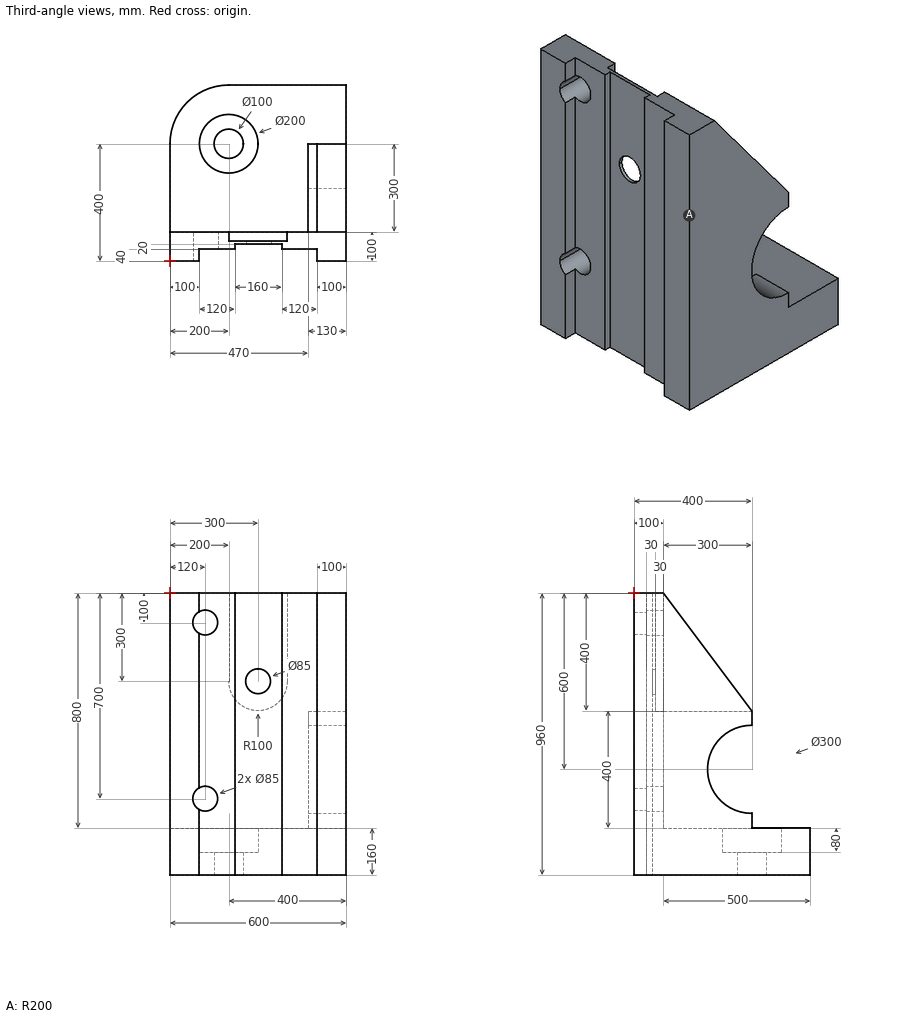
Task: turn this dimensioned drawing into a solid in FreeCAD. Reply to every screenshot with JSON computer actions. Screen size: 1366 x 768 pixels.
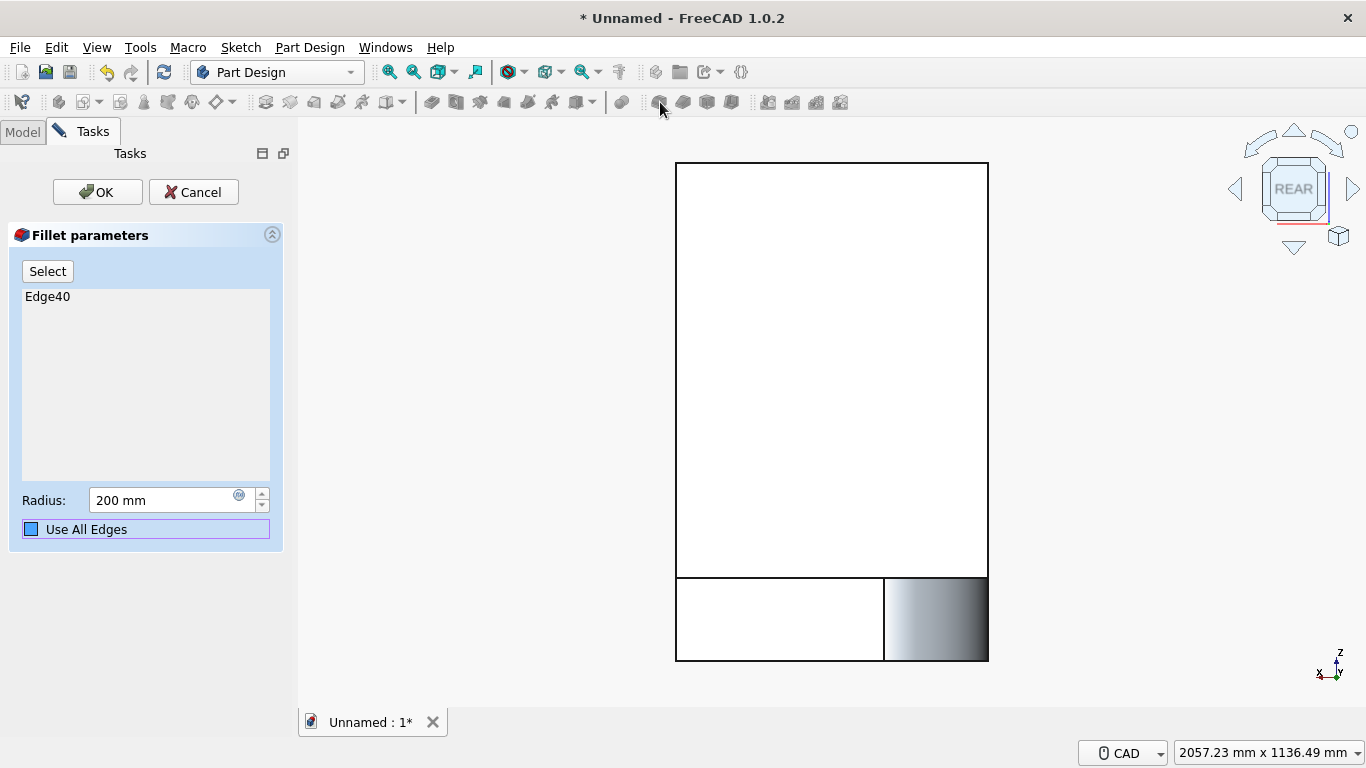
{"action": "left_click", "coordinate": [98, 192]}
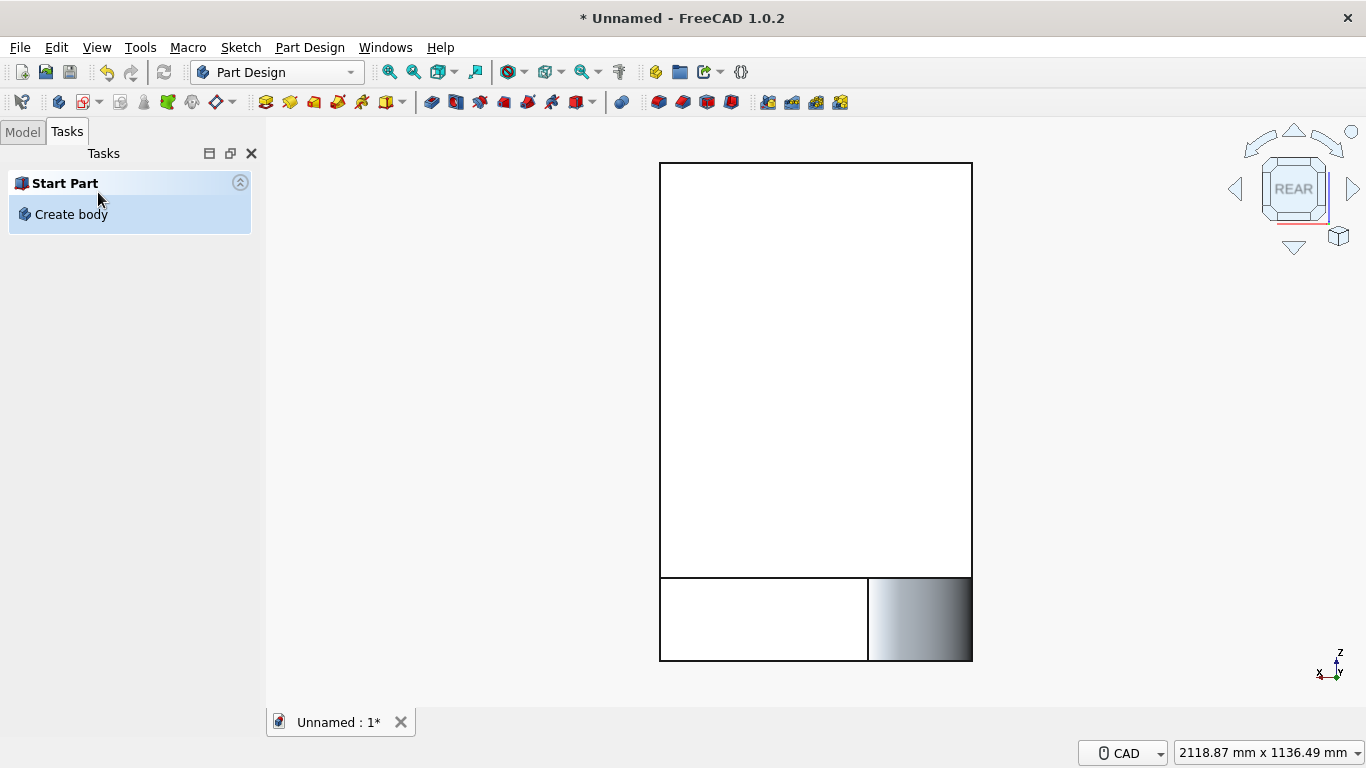
{"action": "key", "text": "0"}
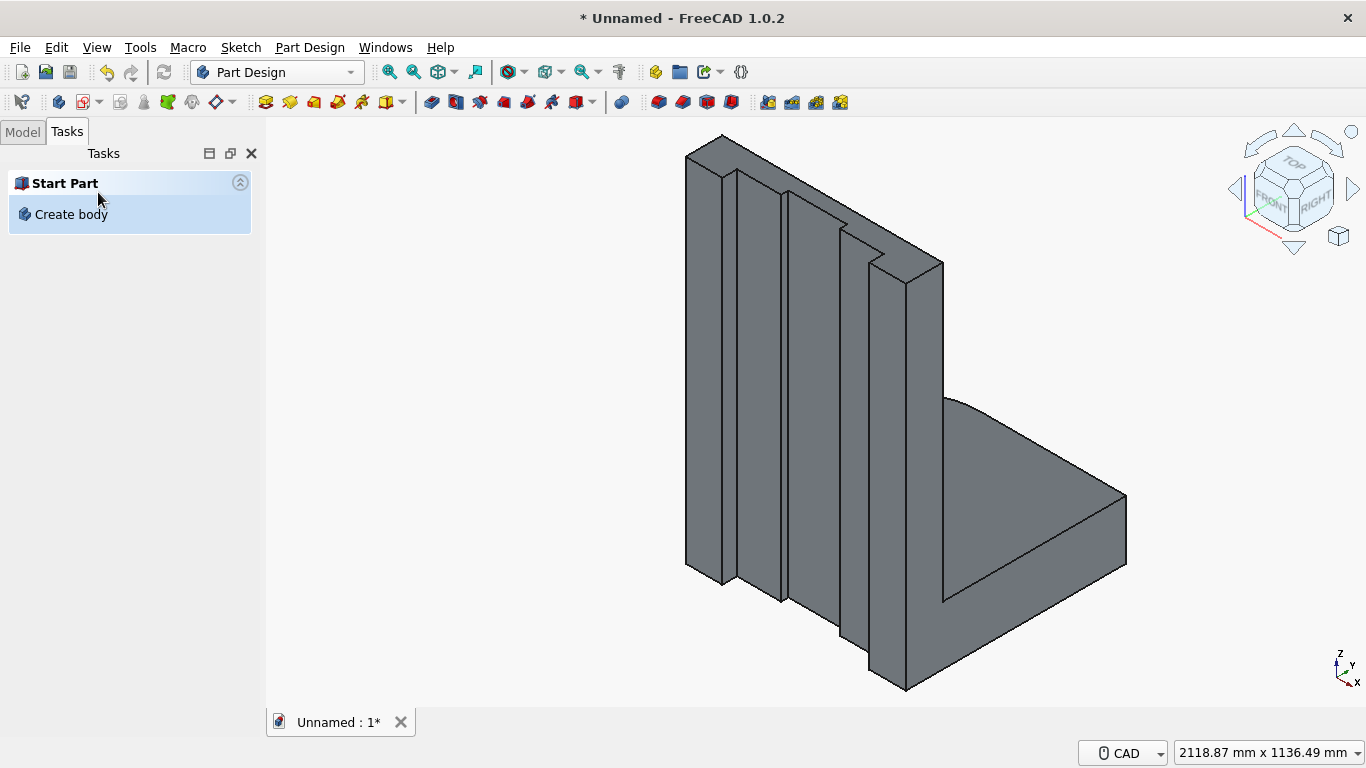
{"action": "left_click", "coordinate": [390, 72]}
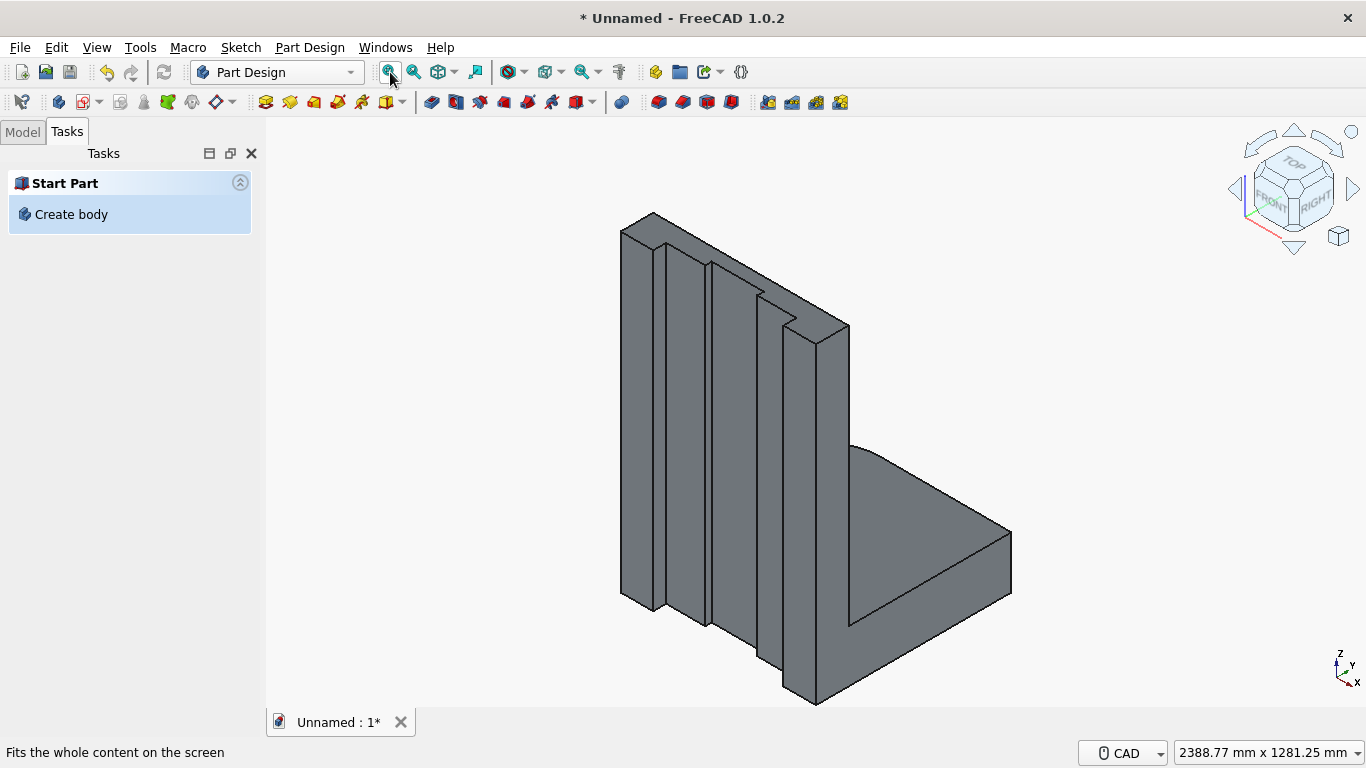
{"action": "left_click", "coordinate": [860, 538]}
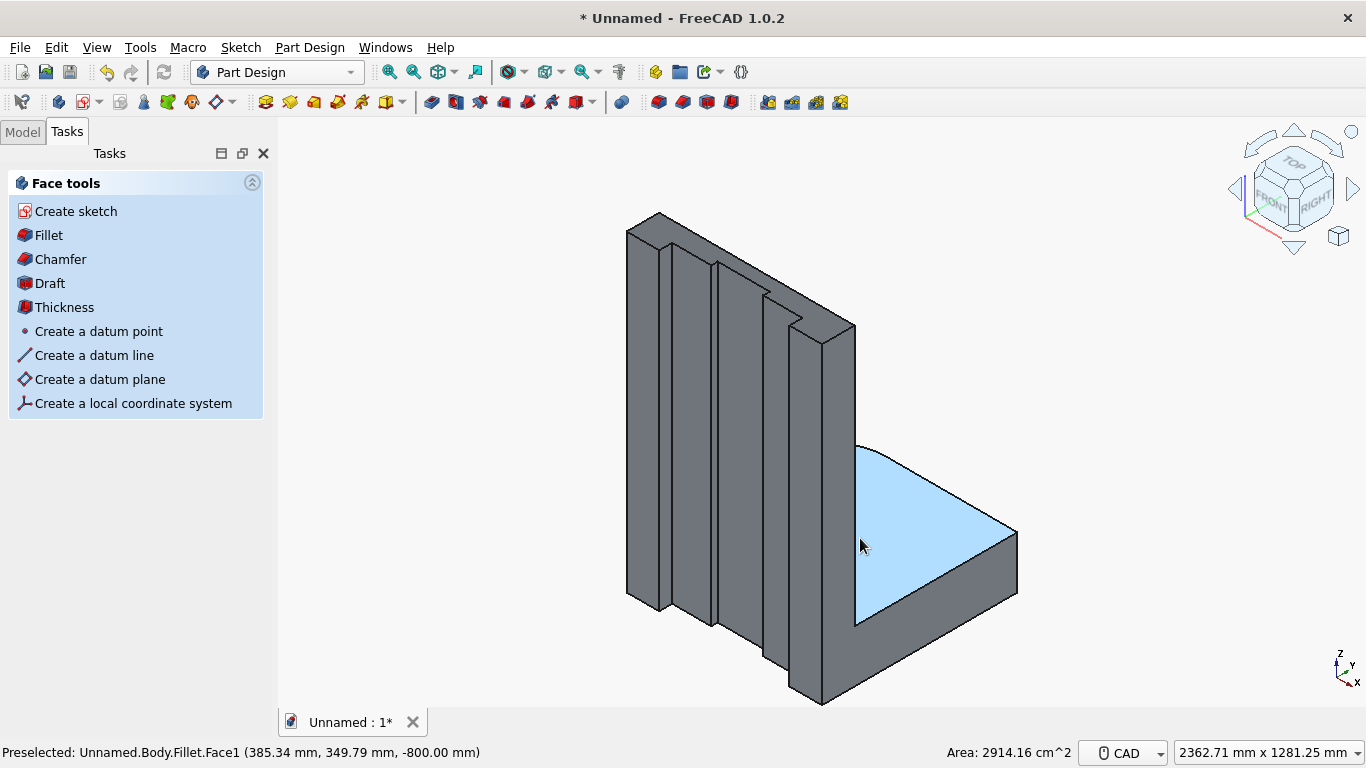
{"action": "left_click", "coordinate": [84, 102]}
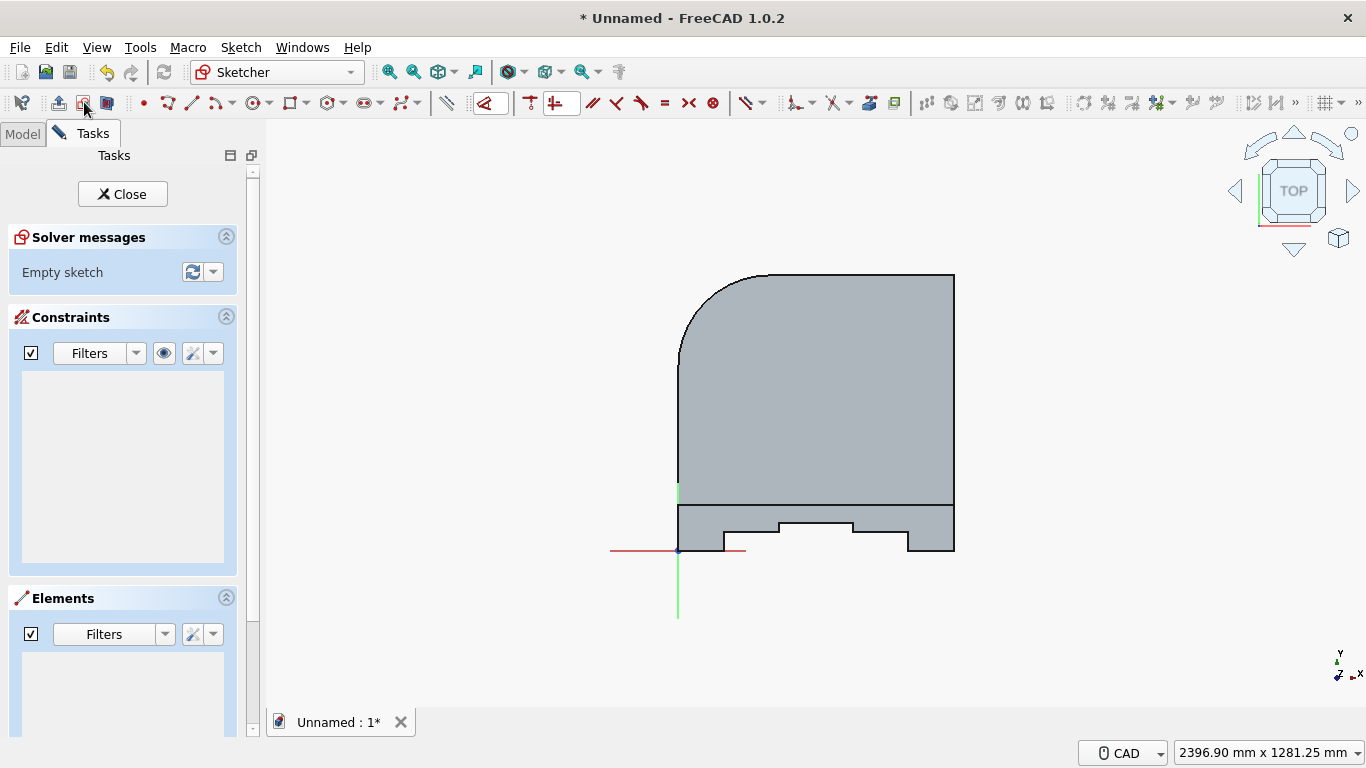
{"action": "scroll", "coordinate": [778, 352], "scroll_direction": "up", "scroll_amount": 7}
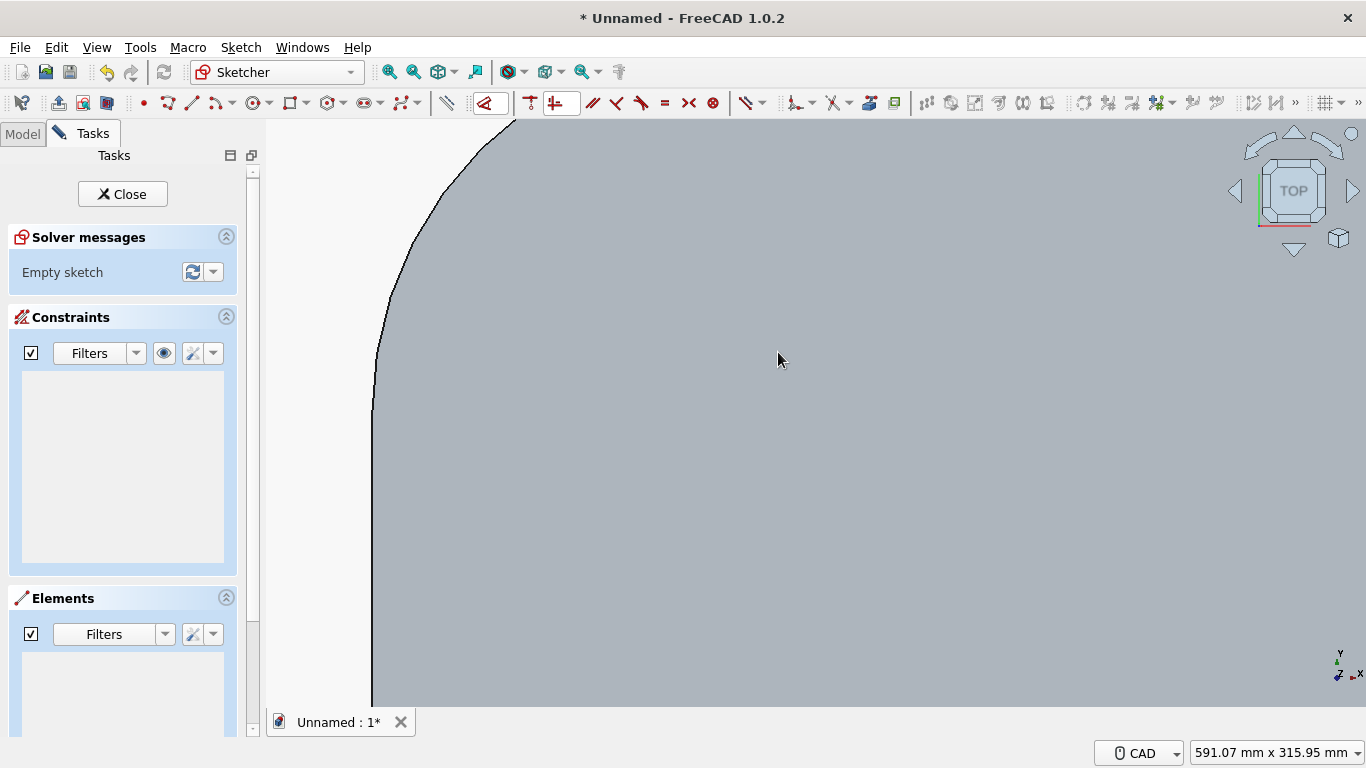
{"action": "left_click", "coordinate": [254, 104]}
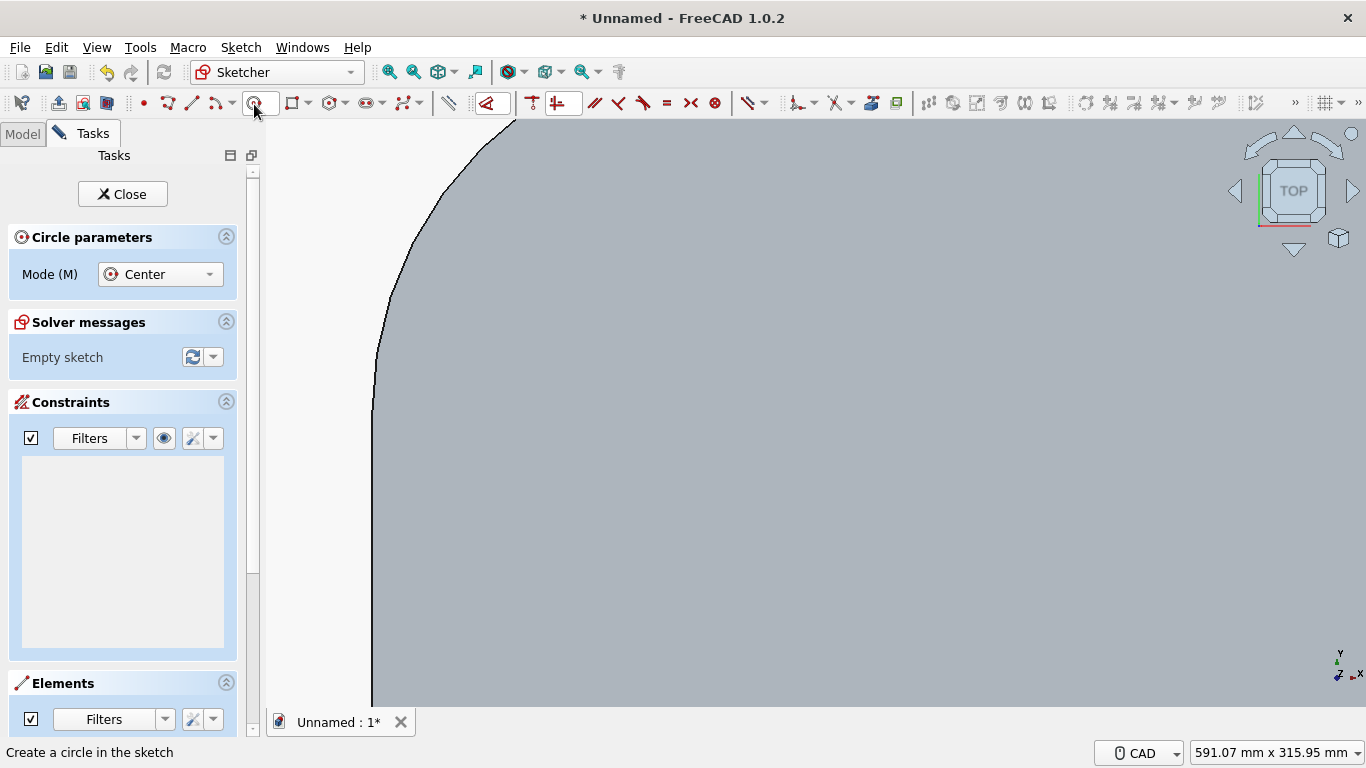
{"action": "left_click", "coordinate": [745, 412]}
{"action": "left_click", "coordinate": [876, 280]}
{"action": "key", "text": "Escape"}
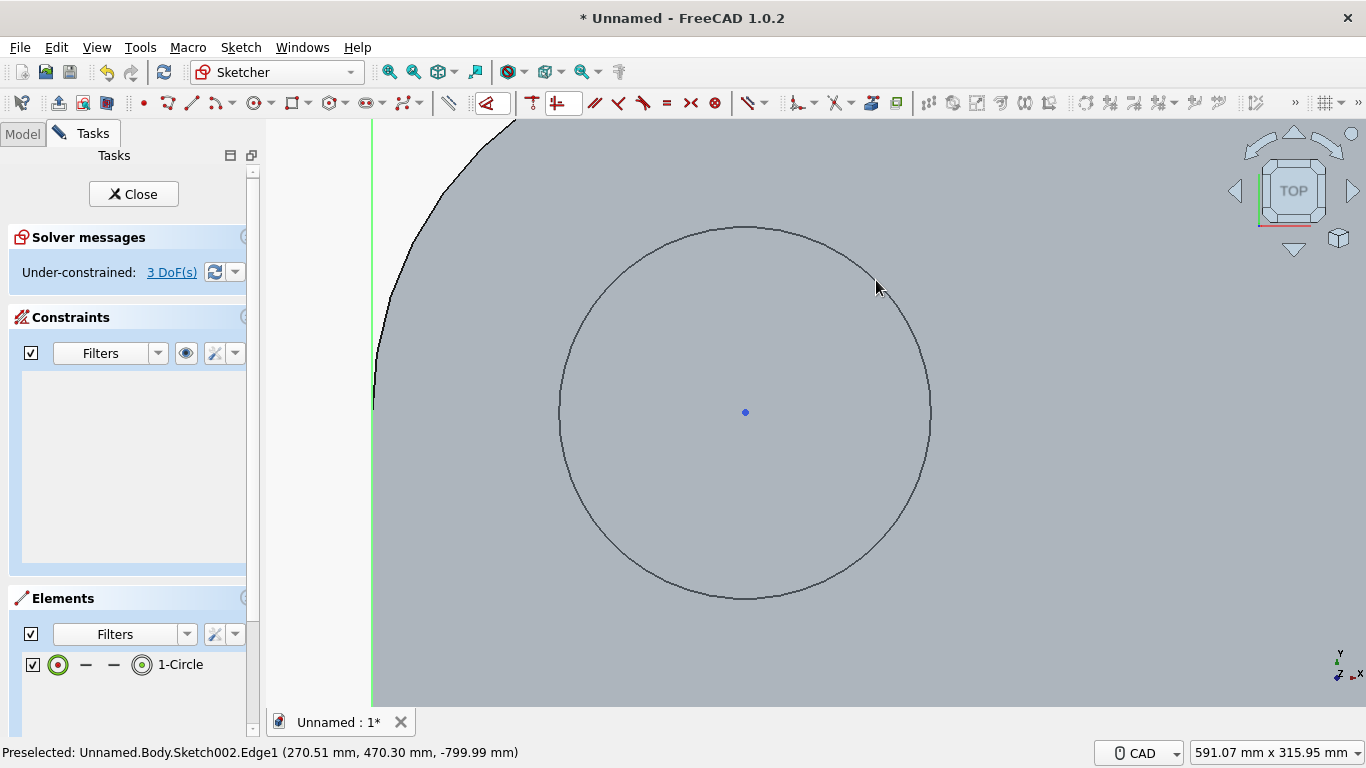
{"action": "left_click", "coordinate": [876, 281]}